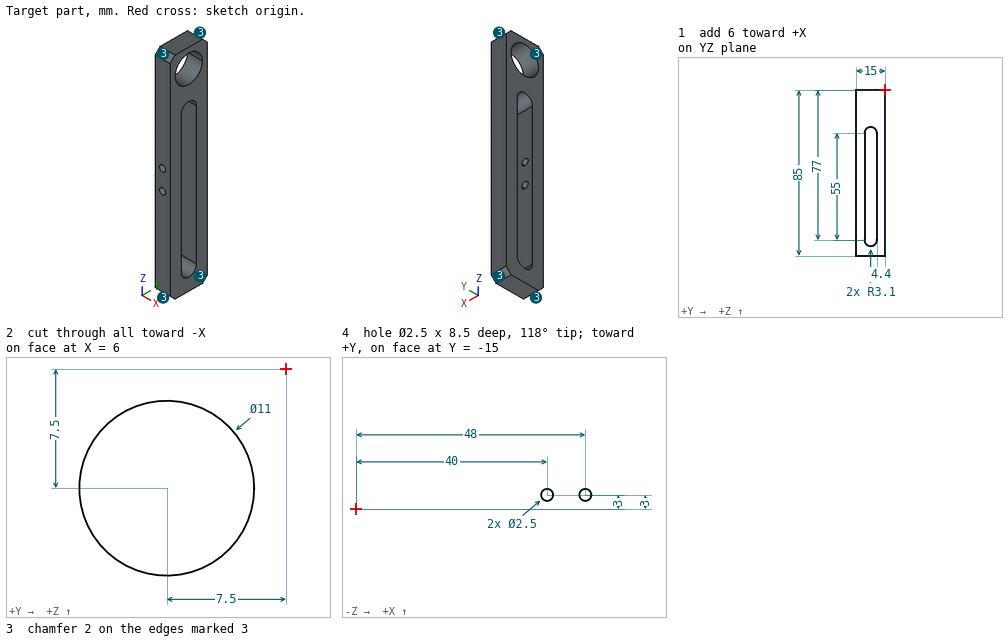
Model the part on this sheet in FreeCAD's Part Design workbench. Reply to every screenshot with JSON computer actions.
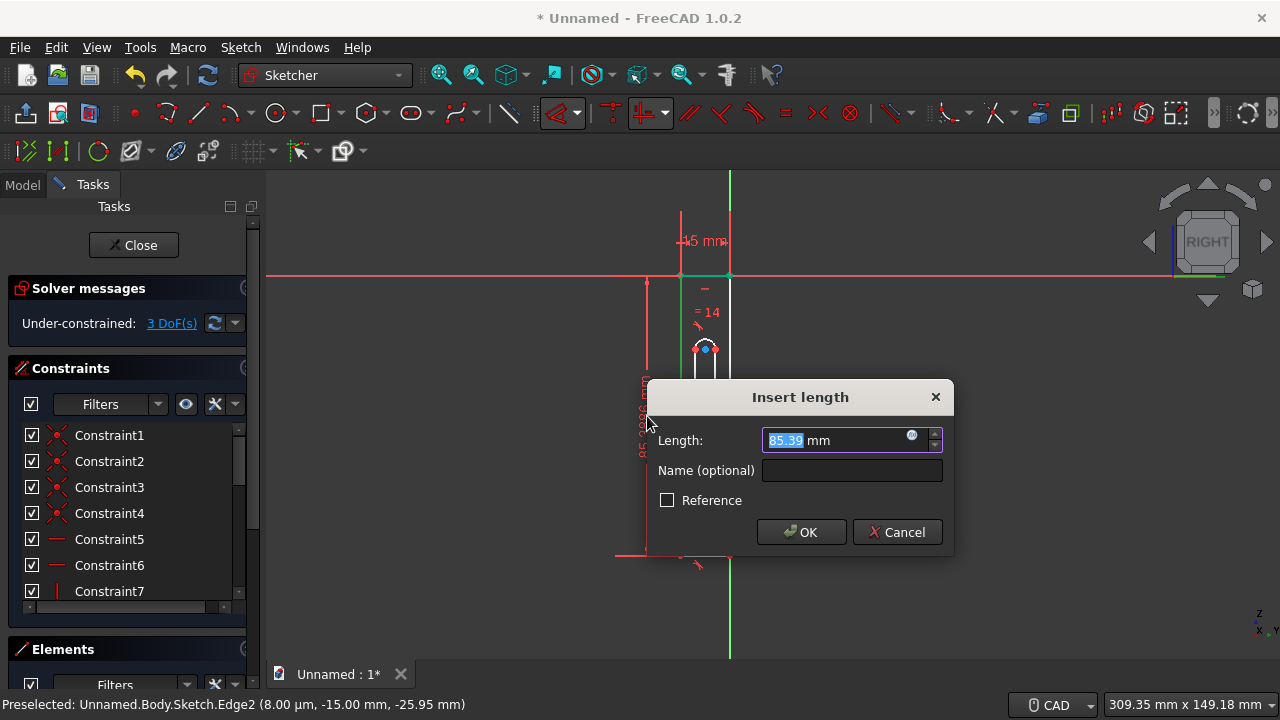
{"action": "type", "text": "85"}
{"action": "key", "text": "Return"}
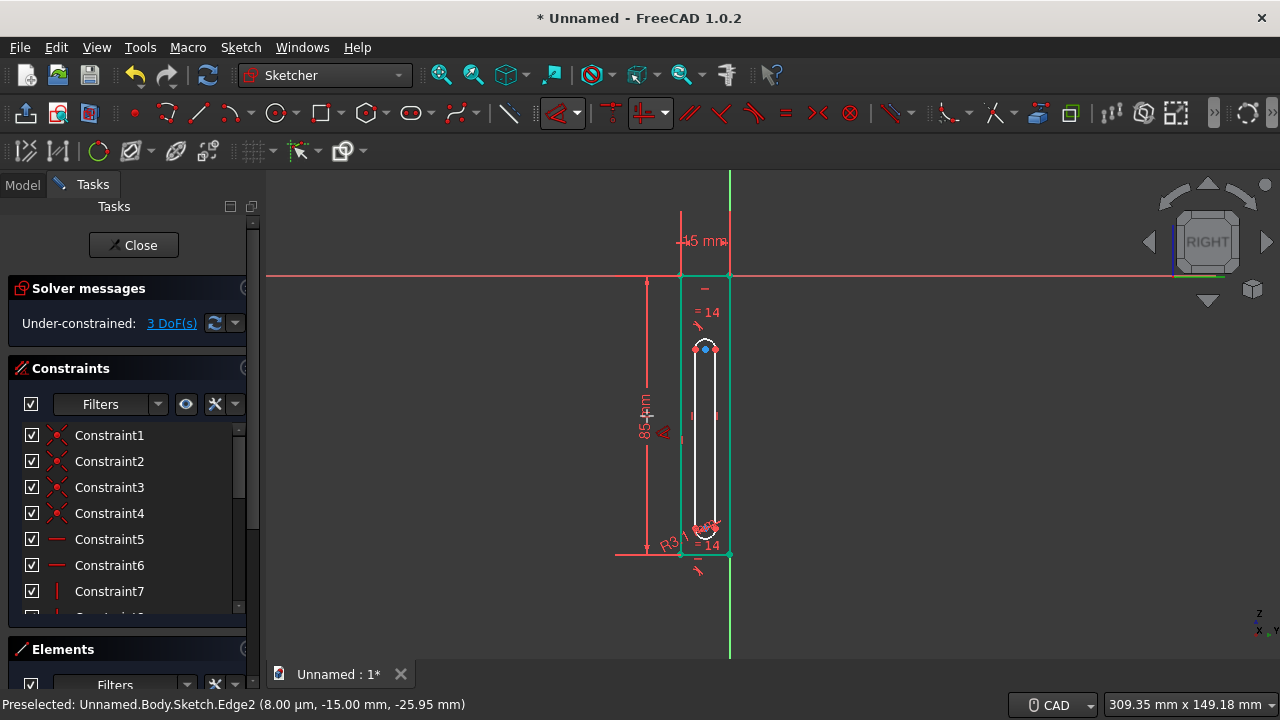
{"action": "left_click", "coordinate": [695, 475]}
{"action": "left_click", "coordinate": [661, 439]}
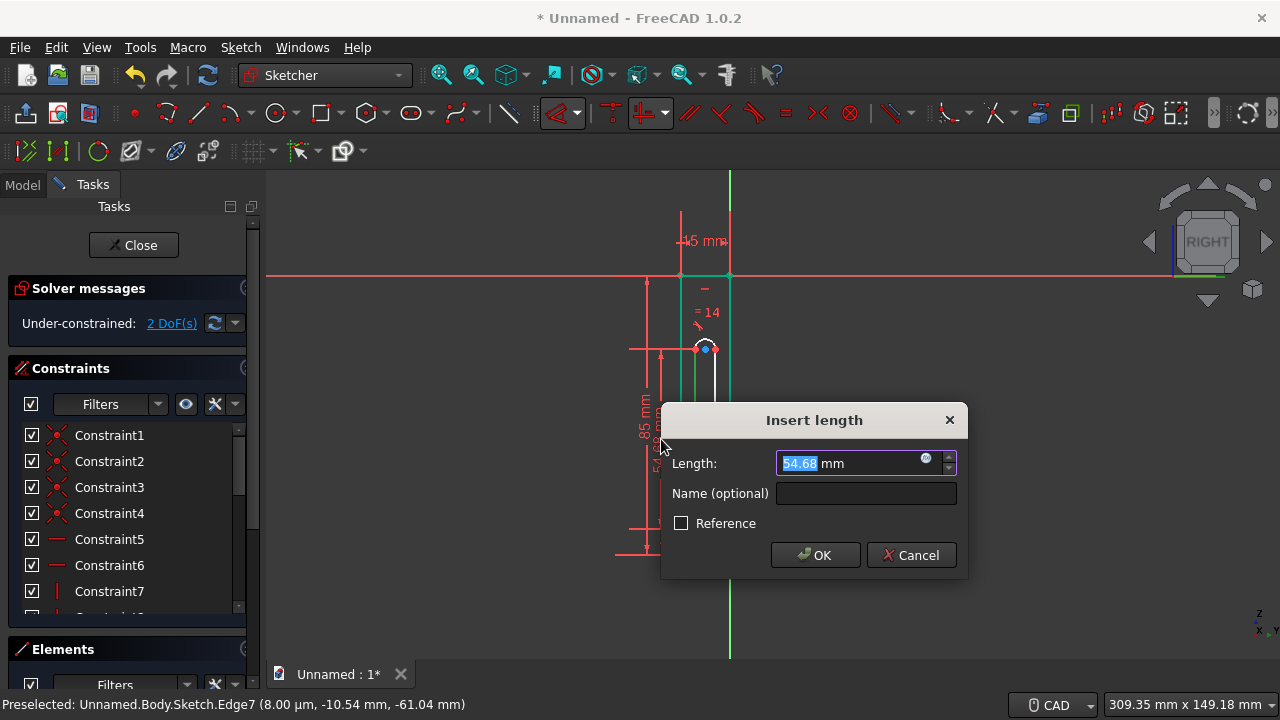
{"action": "type", "text": "55"}
{"action": "key", "text": "Return"}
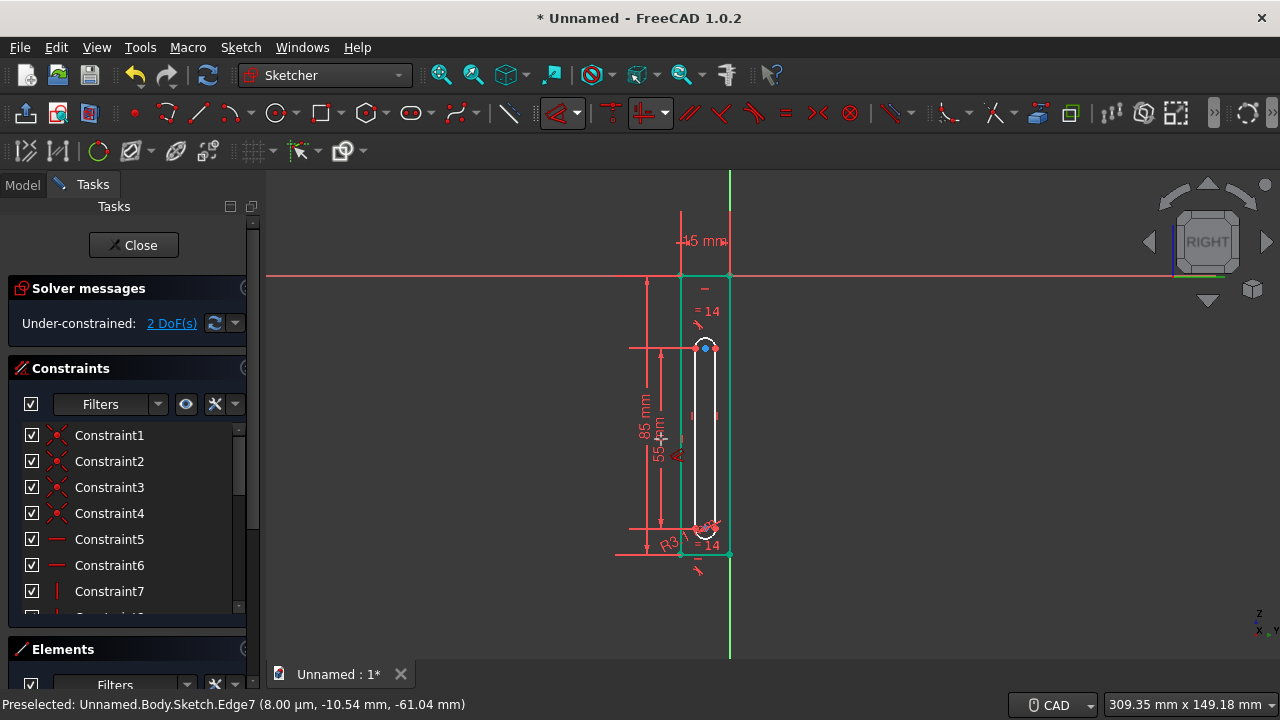
{"action": "left_click", "coordinate": [695, 529]}
{"action": "left_click", "coordinate": [764, 402]}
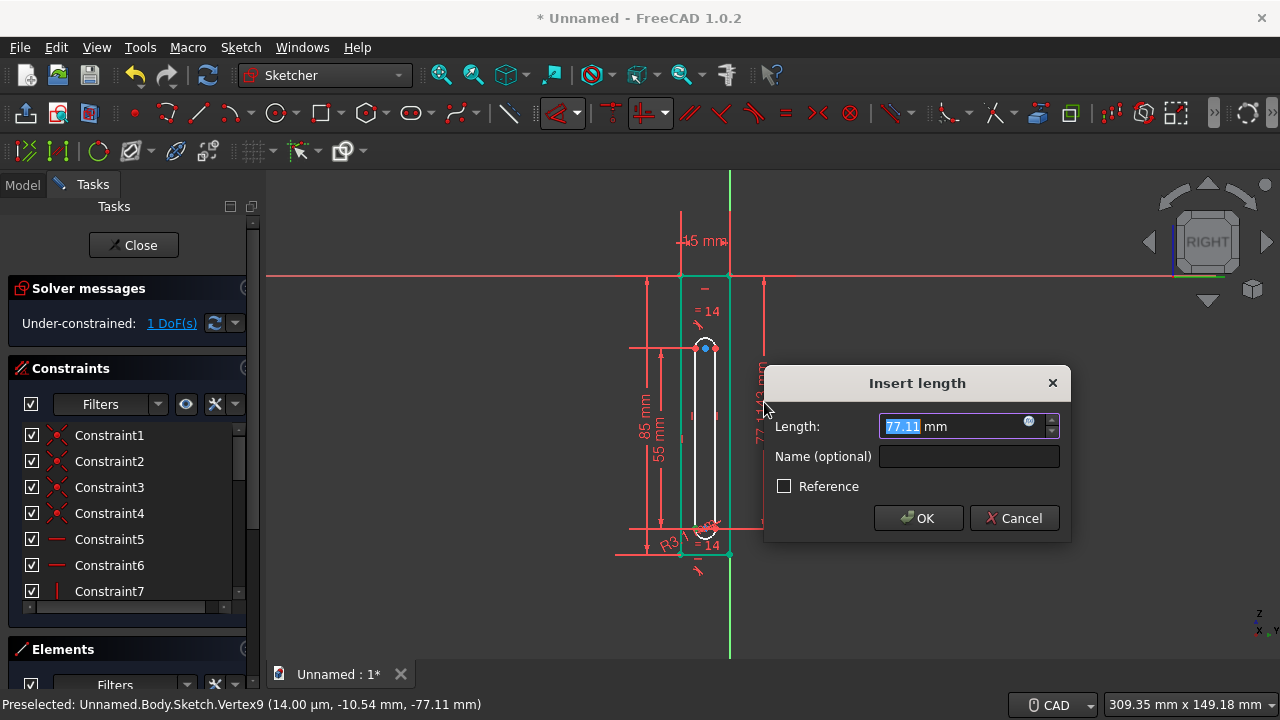
{"action": "type", "text": "77"}
{"action": "key", "text": "Return"}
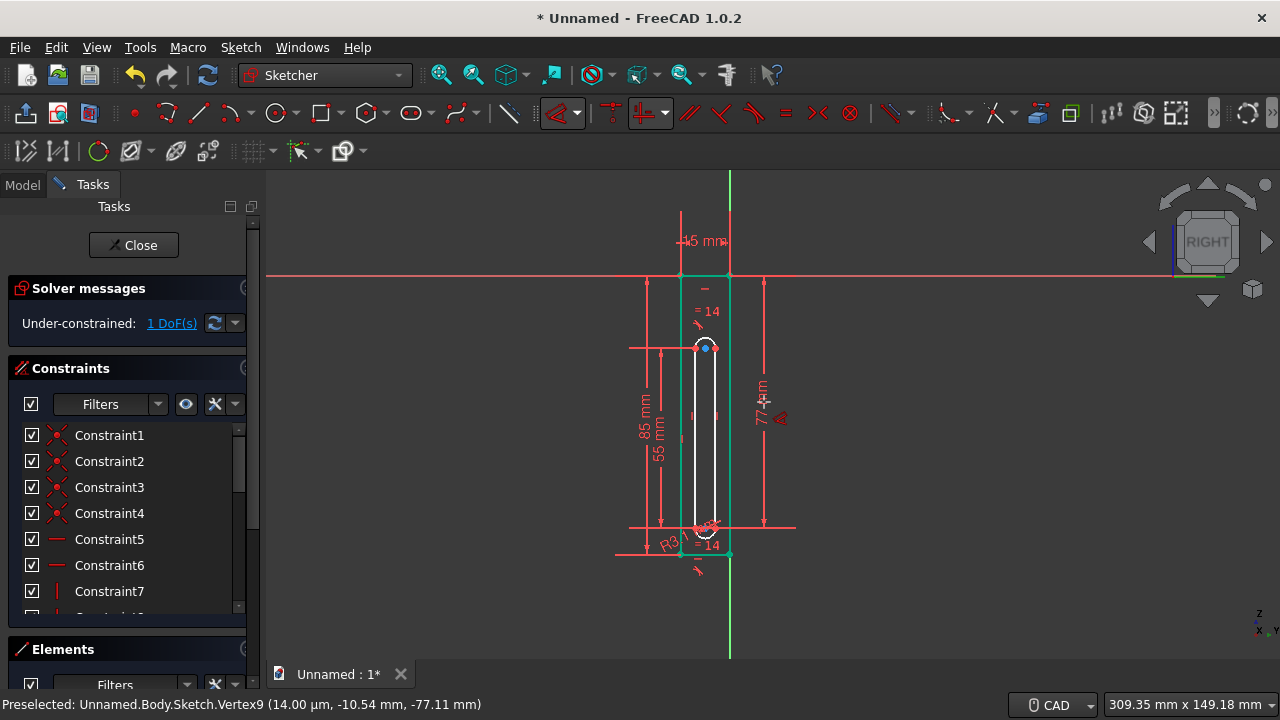
{"action": "scroll", "coordinate": [715, 528], "scroll_direction": "up", "scroll_amount": 6}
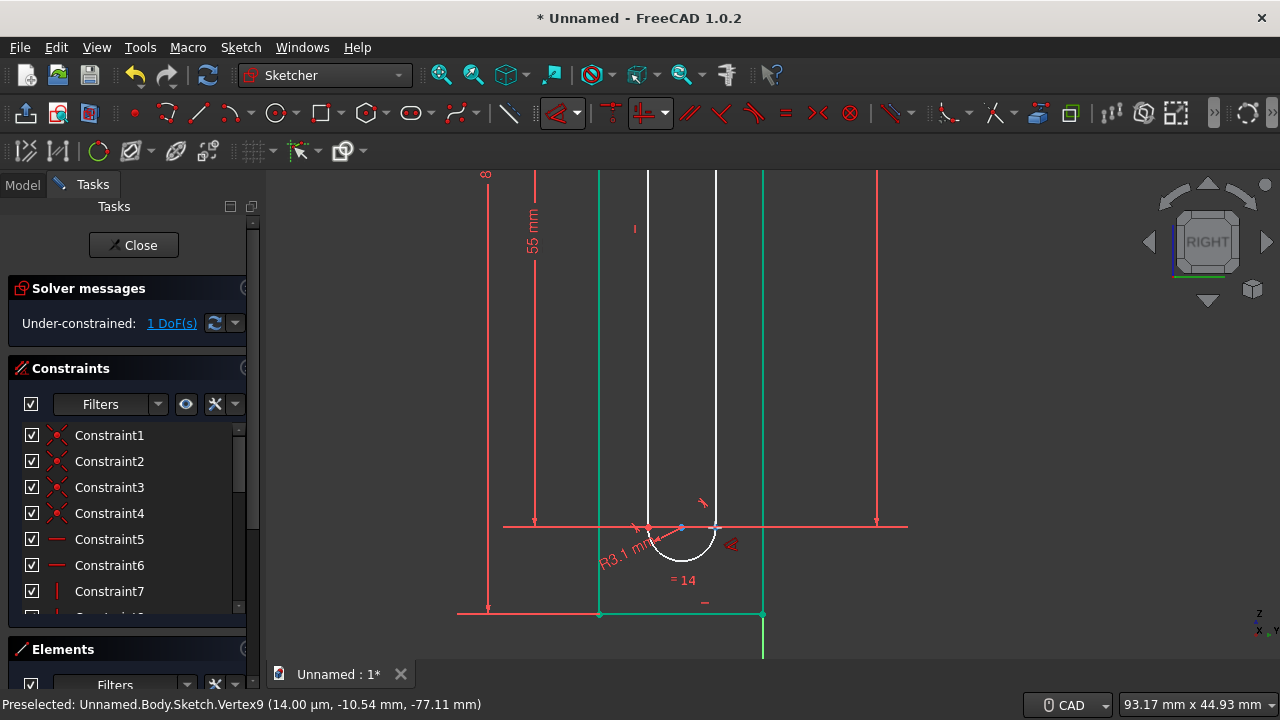
{"action": "left_click", "coordinate": [716, 527]}
{"action": "left_click", "coordinate": [739, 561]}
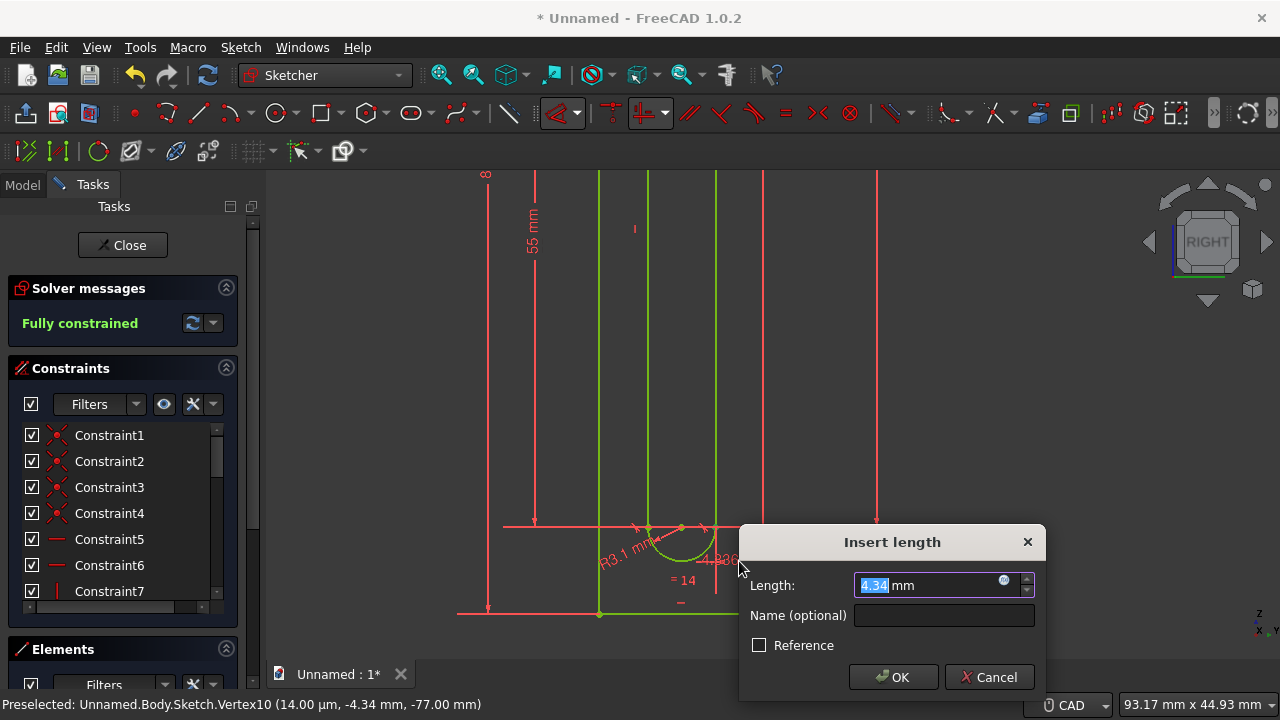
{"action": "type", "text": "4.4"}
{"action": "key", "text": "Return"}
{"action": "key", "text": "Escape"}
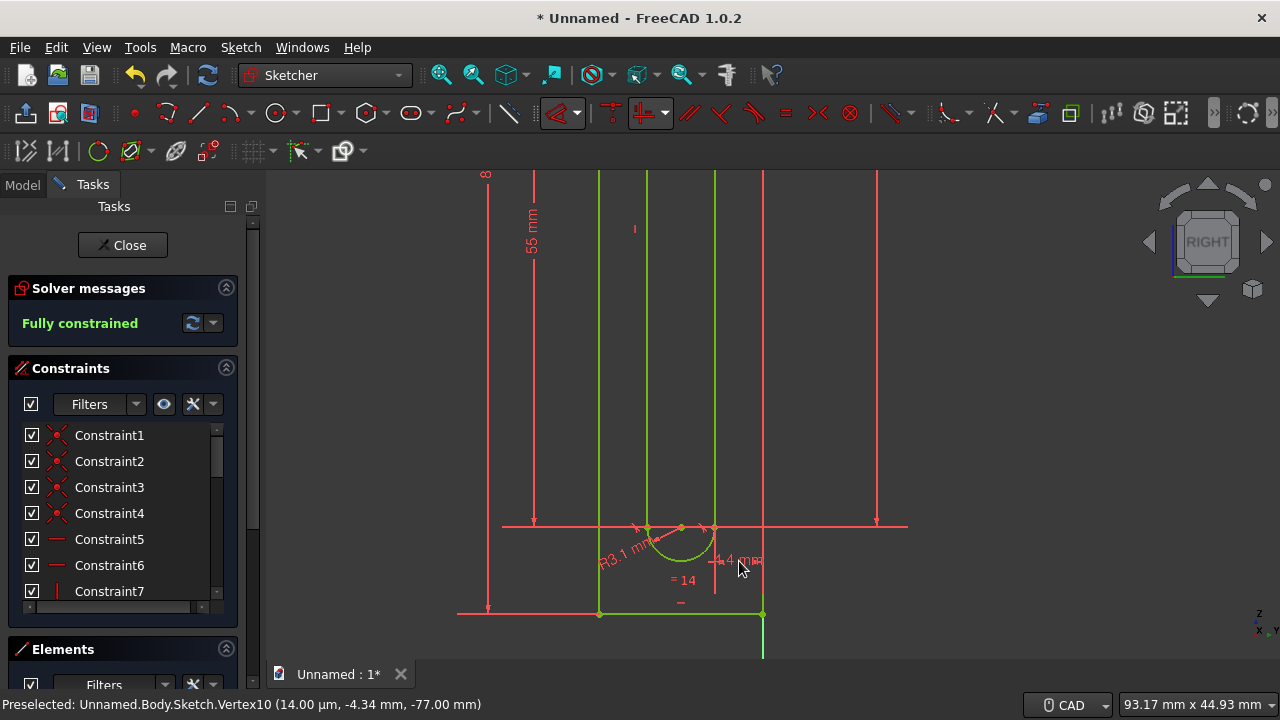
{"action": "left_click", "coordinate": [123, 245]}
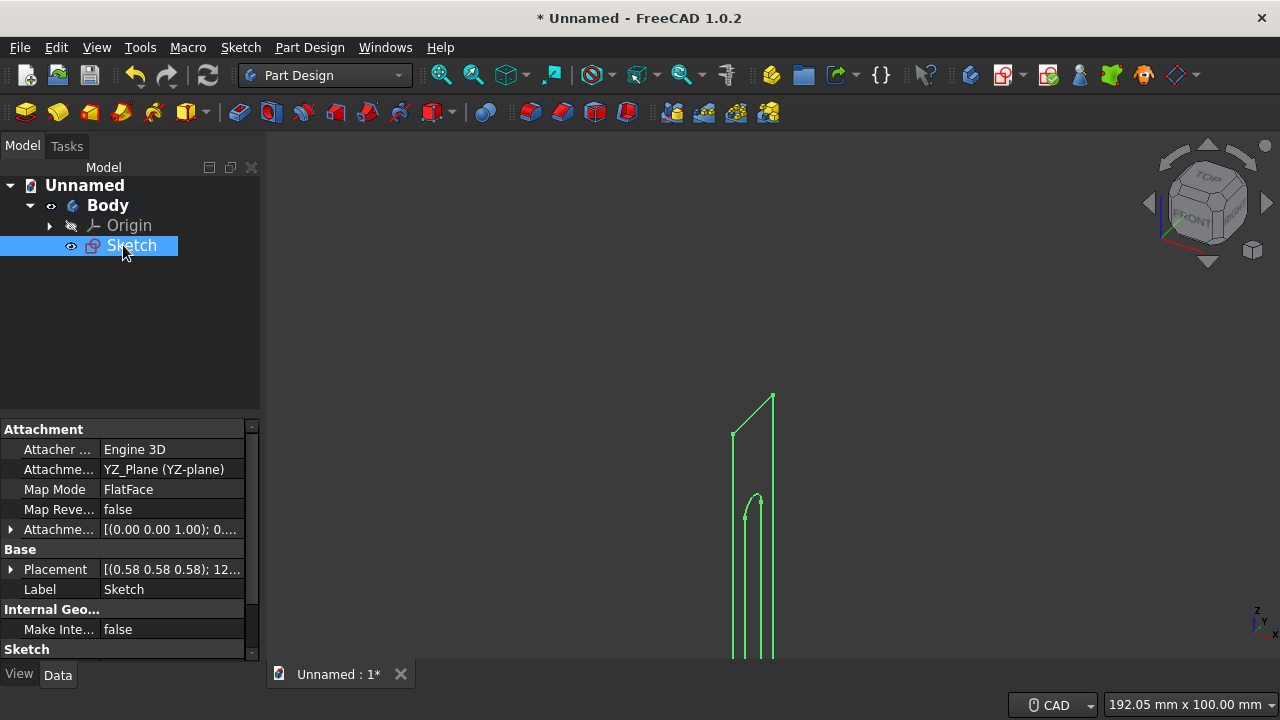
{"action": "left_click", "coordinate": [26, 112]}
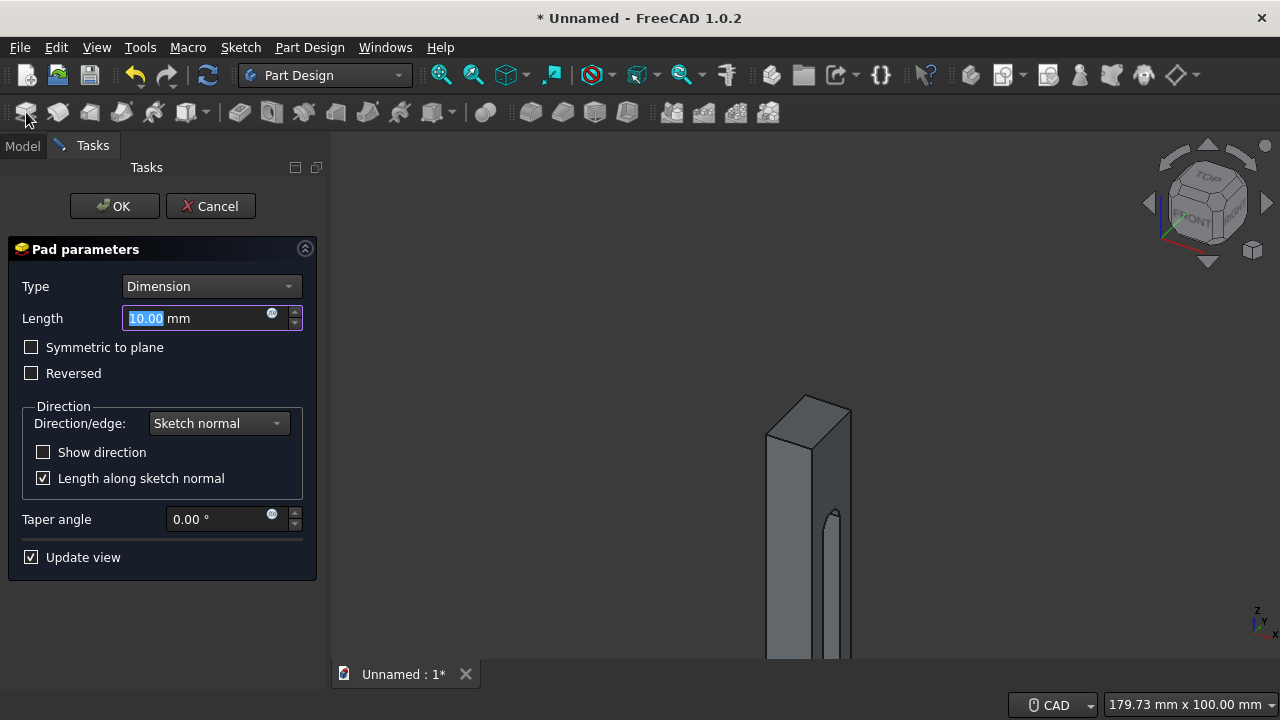
{"action": "type", "text": "6"}
{"action": "key", "text": "Tab"}